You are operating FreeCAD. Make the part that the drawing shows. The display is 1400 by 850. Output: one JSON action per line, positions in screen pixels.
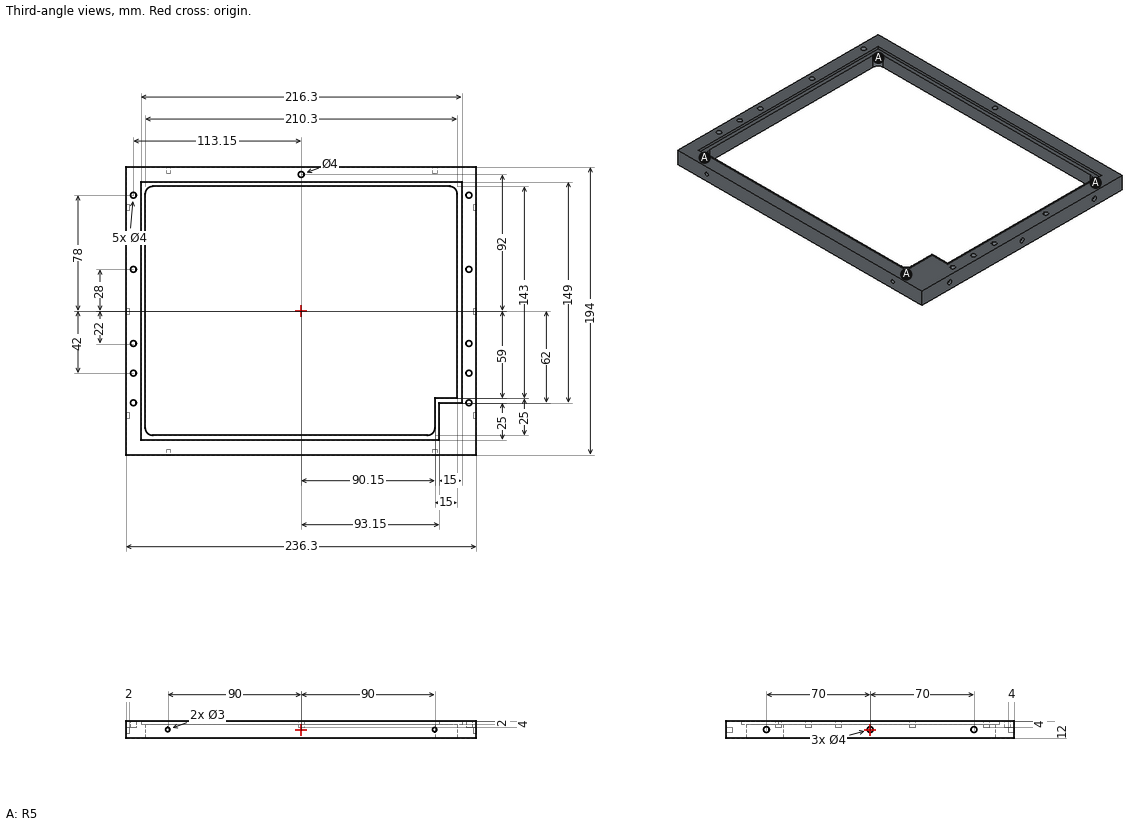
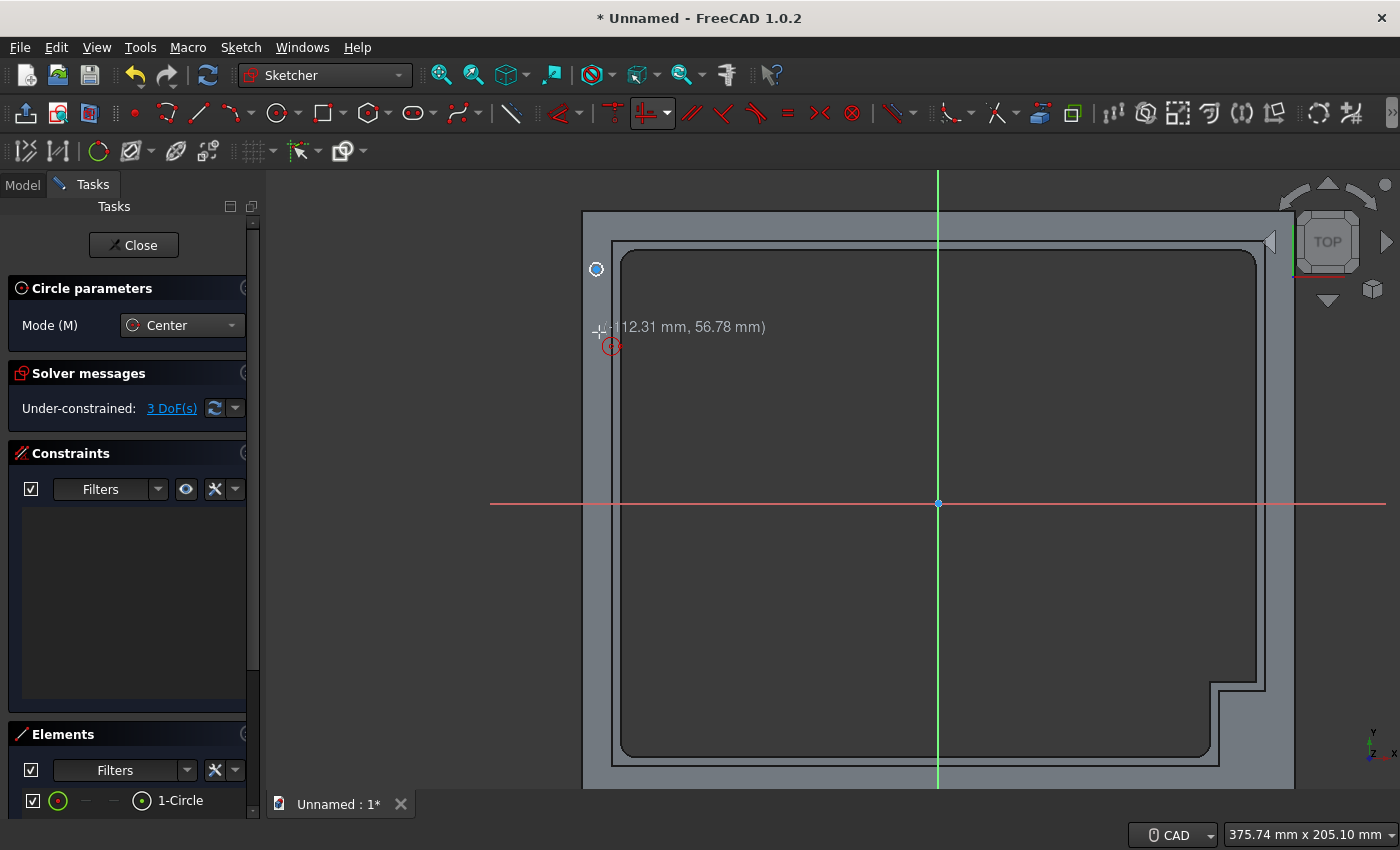
{"action": "left_click", "coordinate": [597, 419]}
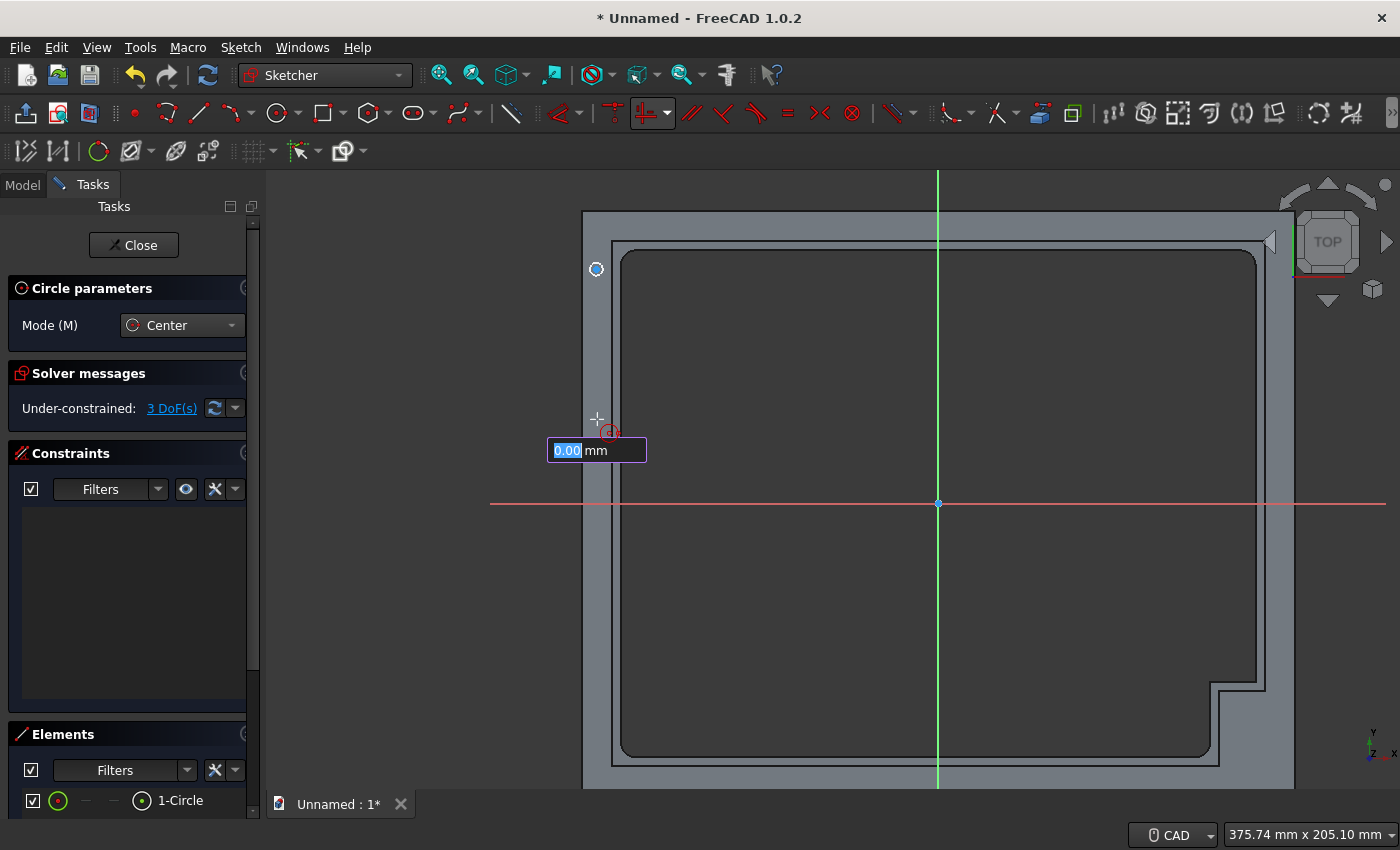
{"action": "scroll", "coordinate": [601, 415], "scroll_direction": "up", "scroll_amount": 5}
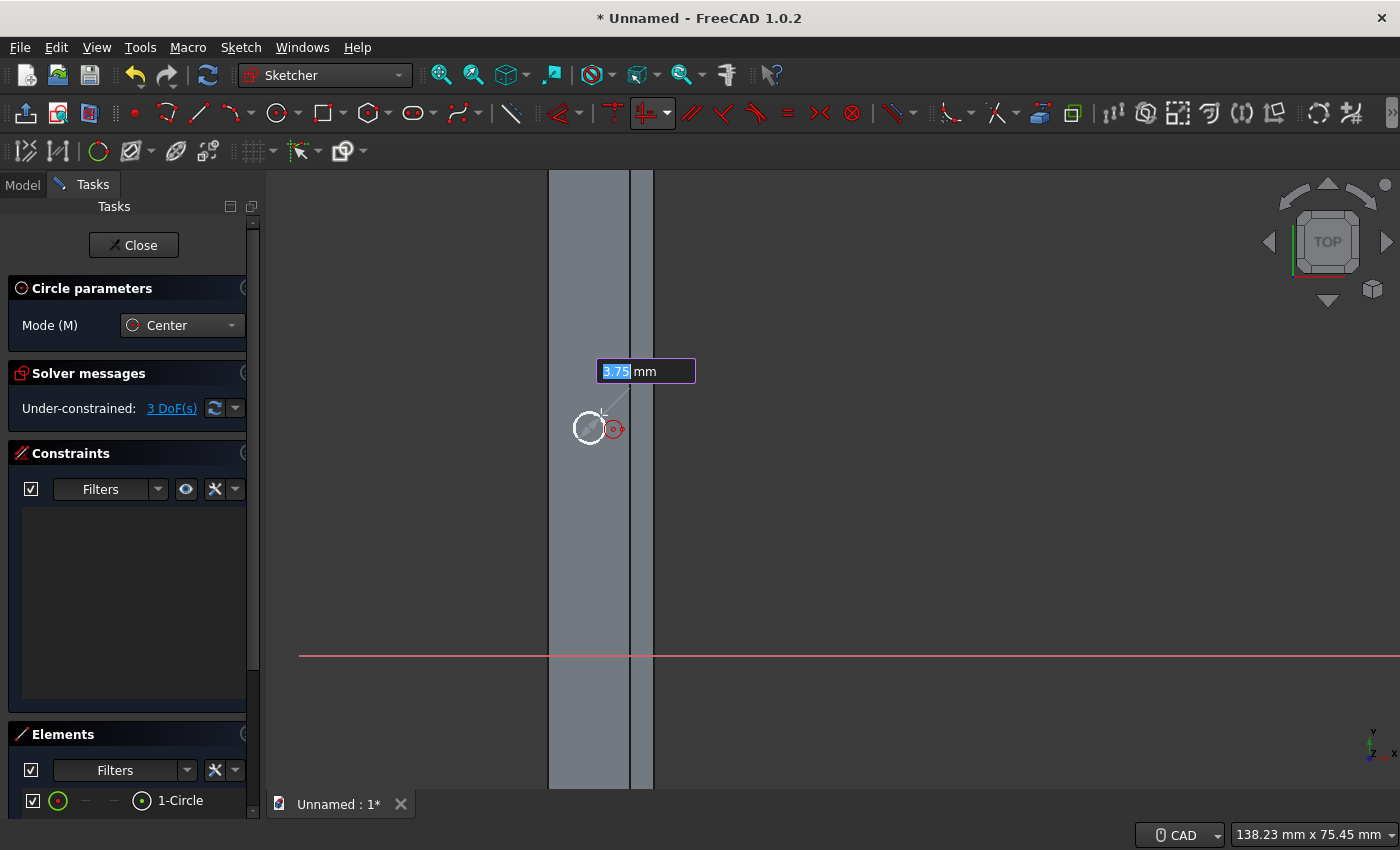
{"action": "left_click", "coordinate": [600, 414]}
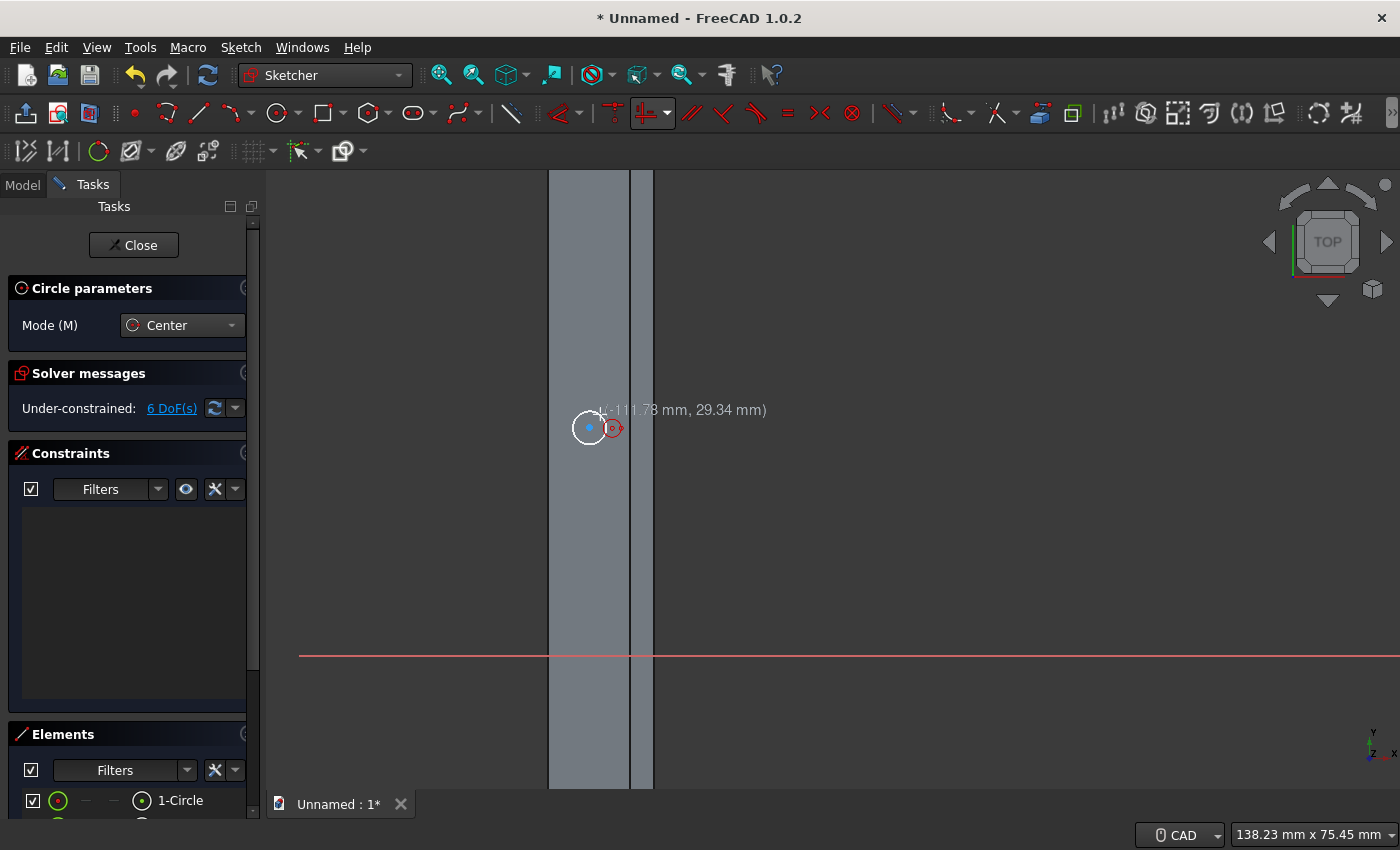
{"action": "scroll", "coordinate": [601, 415], "scroll_direction": "down", "scroll_amount": 5}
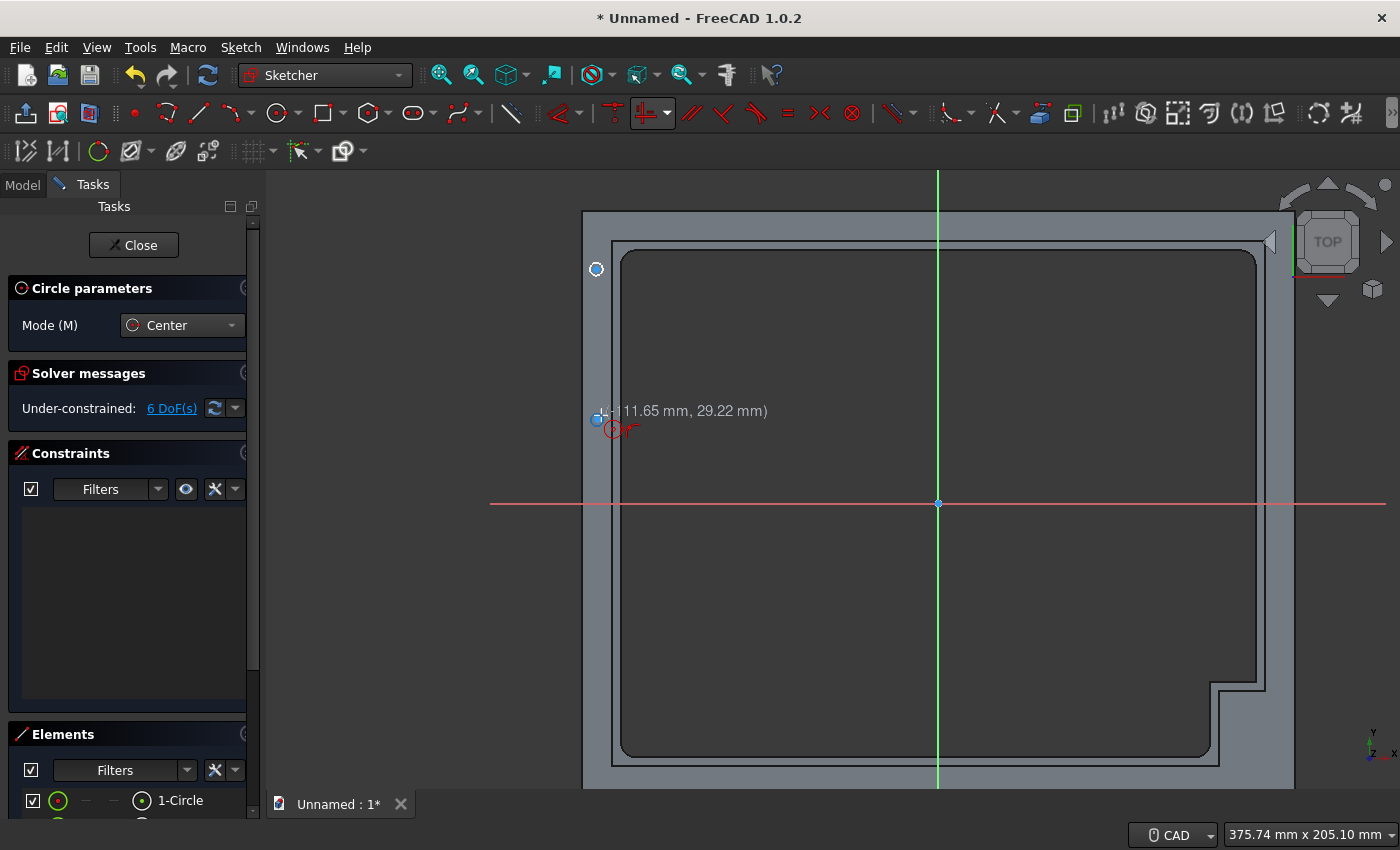
{"action": "scroll", "coordinate": [597, 570], "scroll_direction": "up", "scroll_amount": 7}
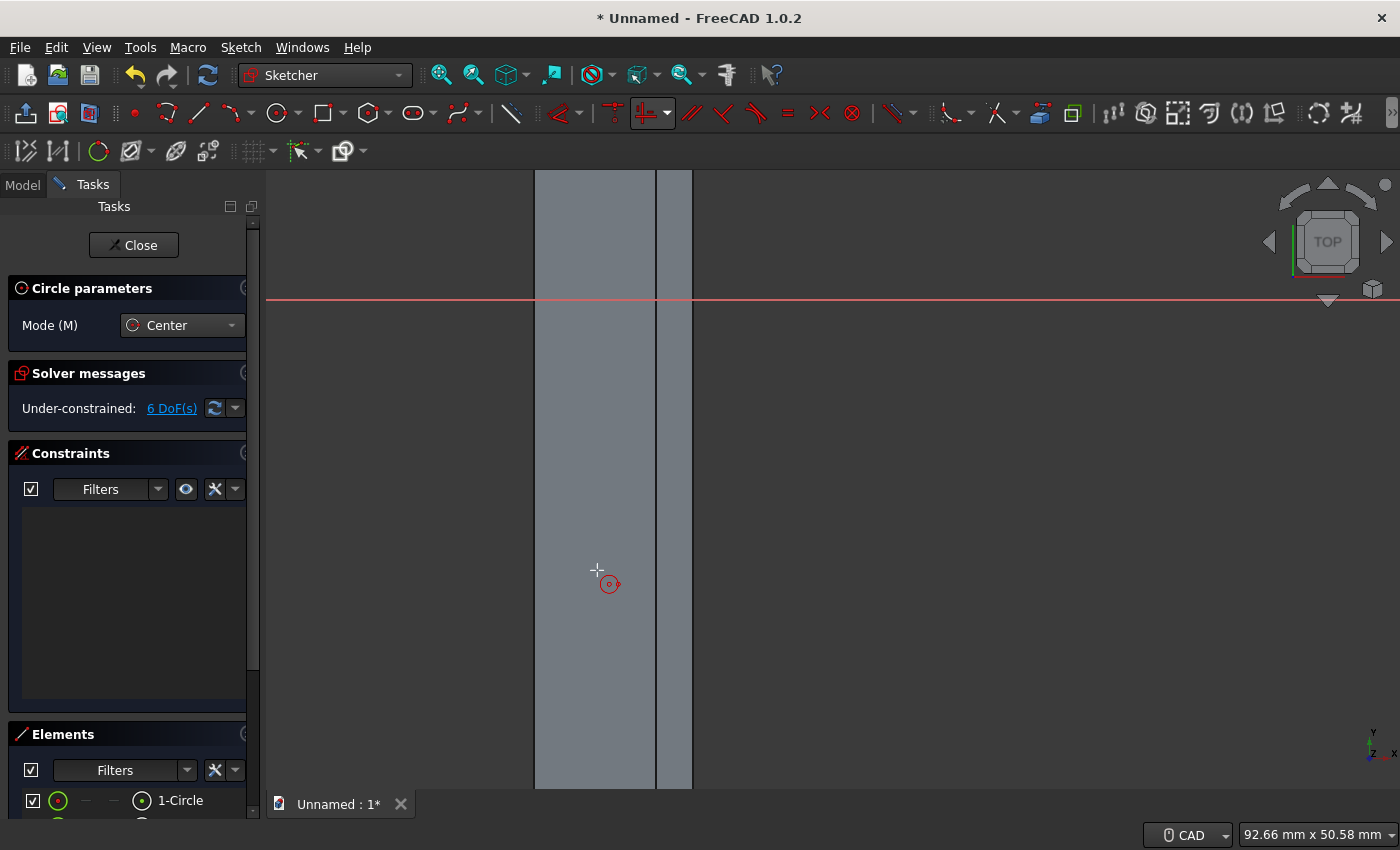
{"action": "scroll", "coordinate": [597, 570], "scroll_direction": "down", "scroll_amount": 7}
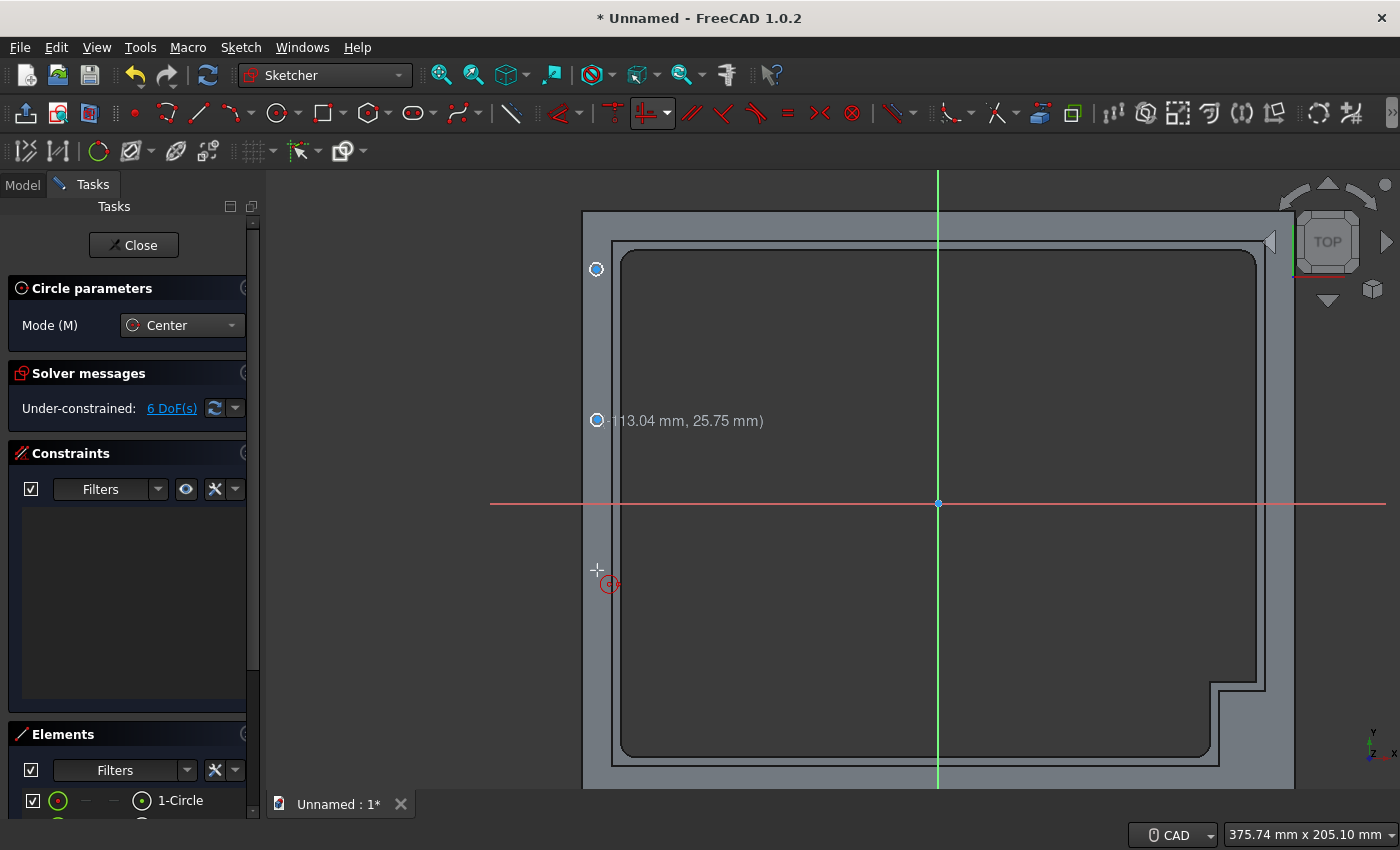
{"action": "left_click", "coordinate": [597, 570]}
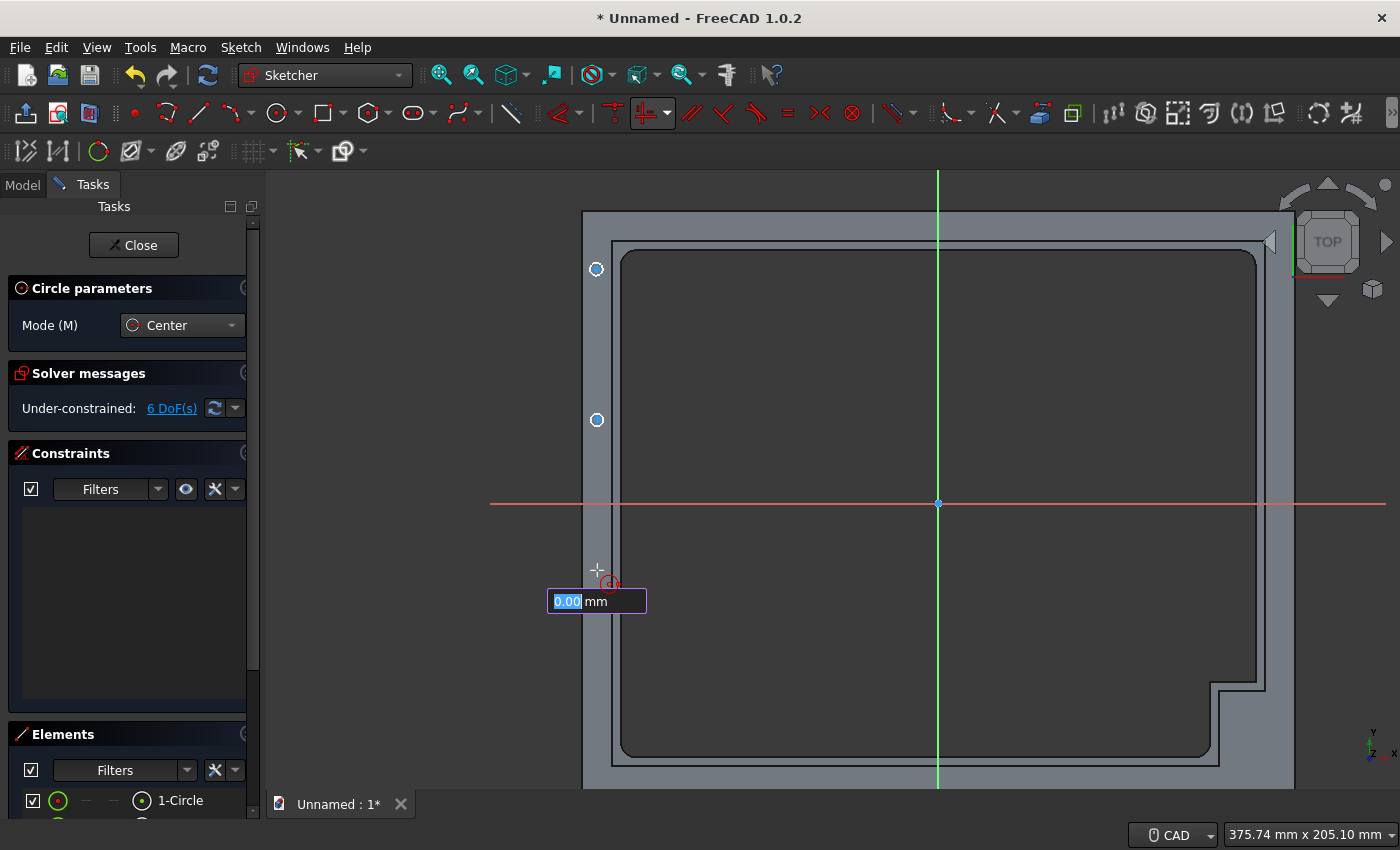
{"action": "scroll", "coordinate": [601, 566], "scroll_direction": "up", "scroll_amount": 5}